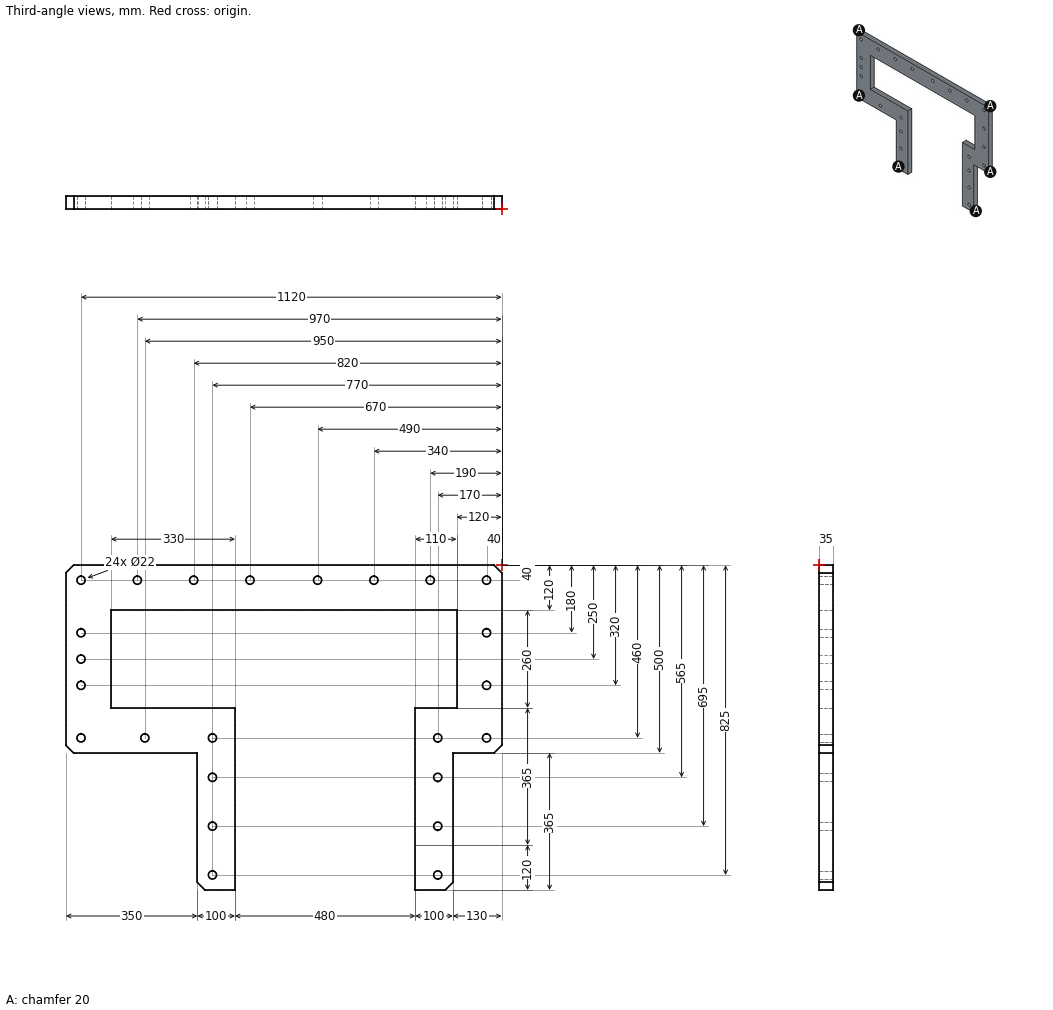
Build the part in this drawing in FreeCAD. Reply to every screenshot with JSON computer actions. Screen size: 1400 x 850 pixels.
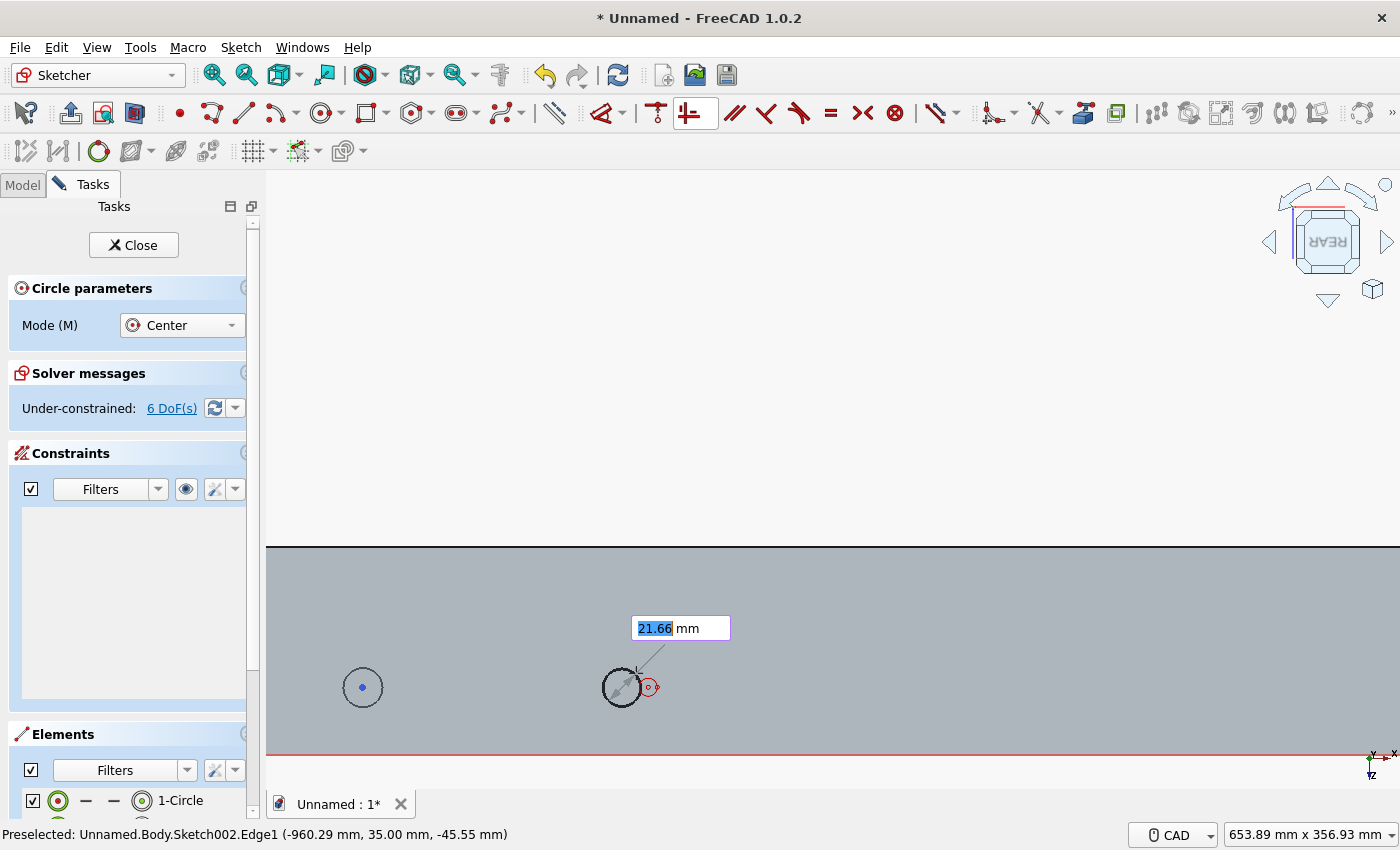
{"action": "left_click", "coordinate": [636, 672]}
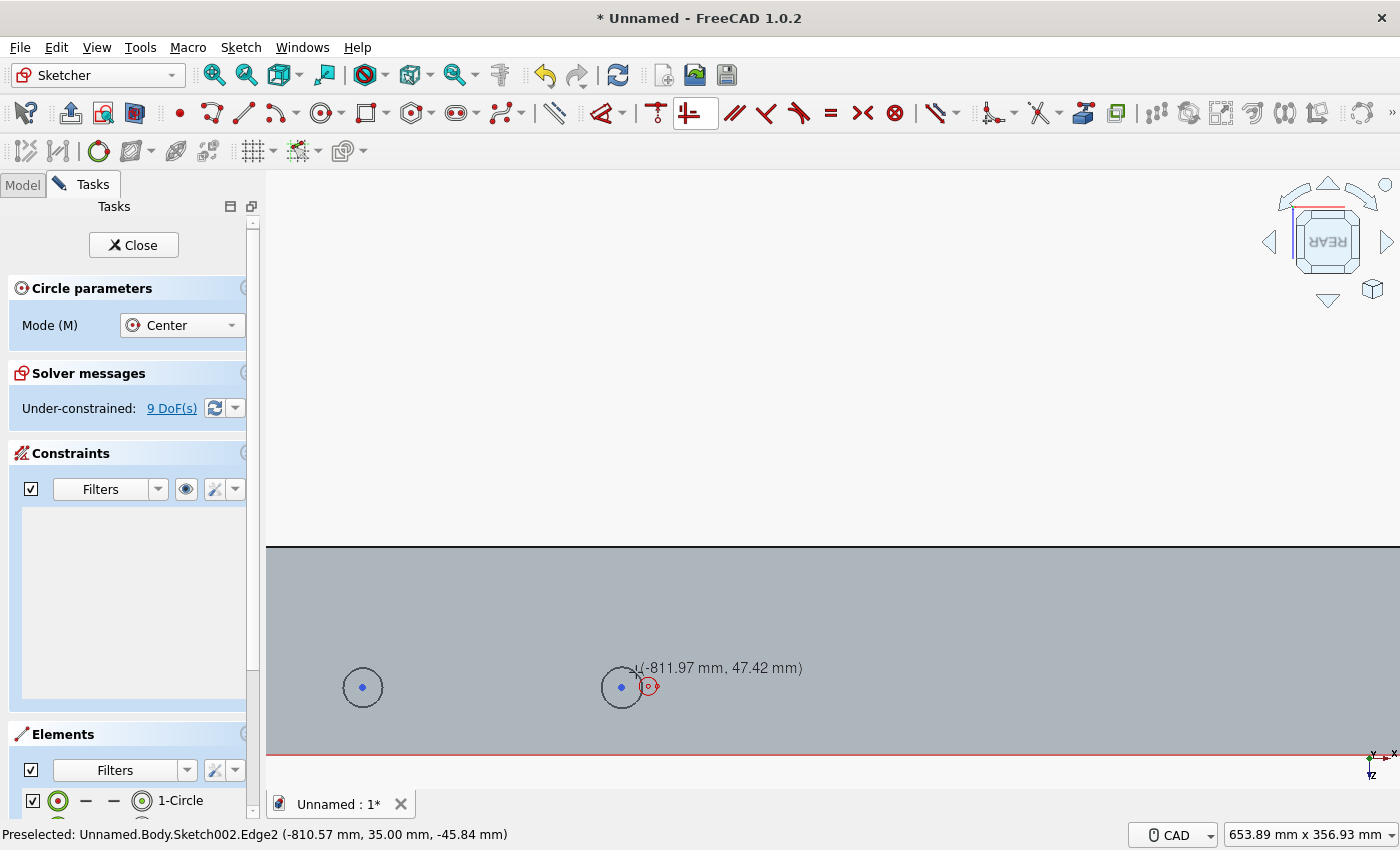
{"action": "scroll", "coordinate": [636, 673], "scroll_direction": "down", "scroll_amount": 6}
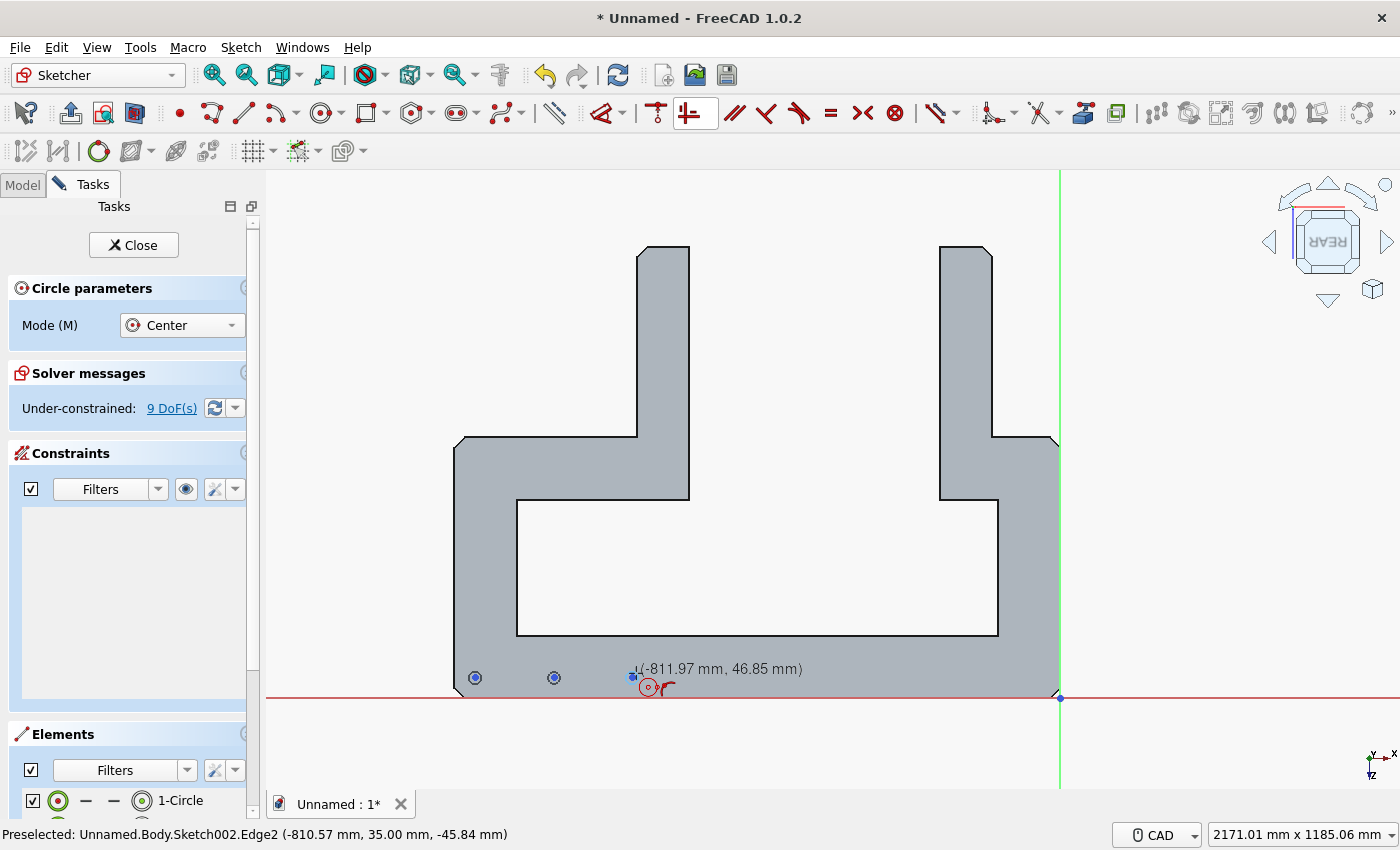
{"action": "left_click", "coordinate": [710, 677]}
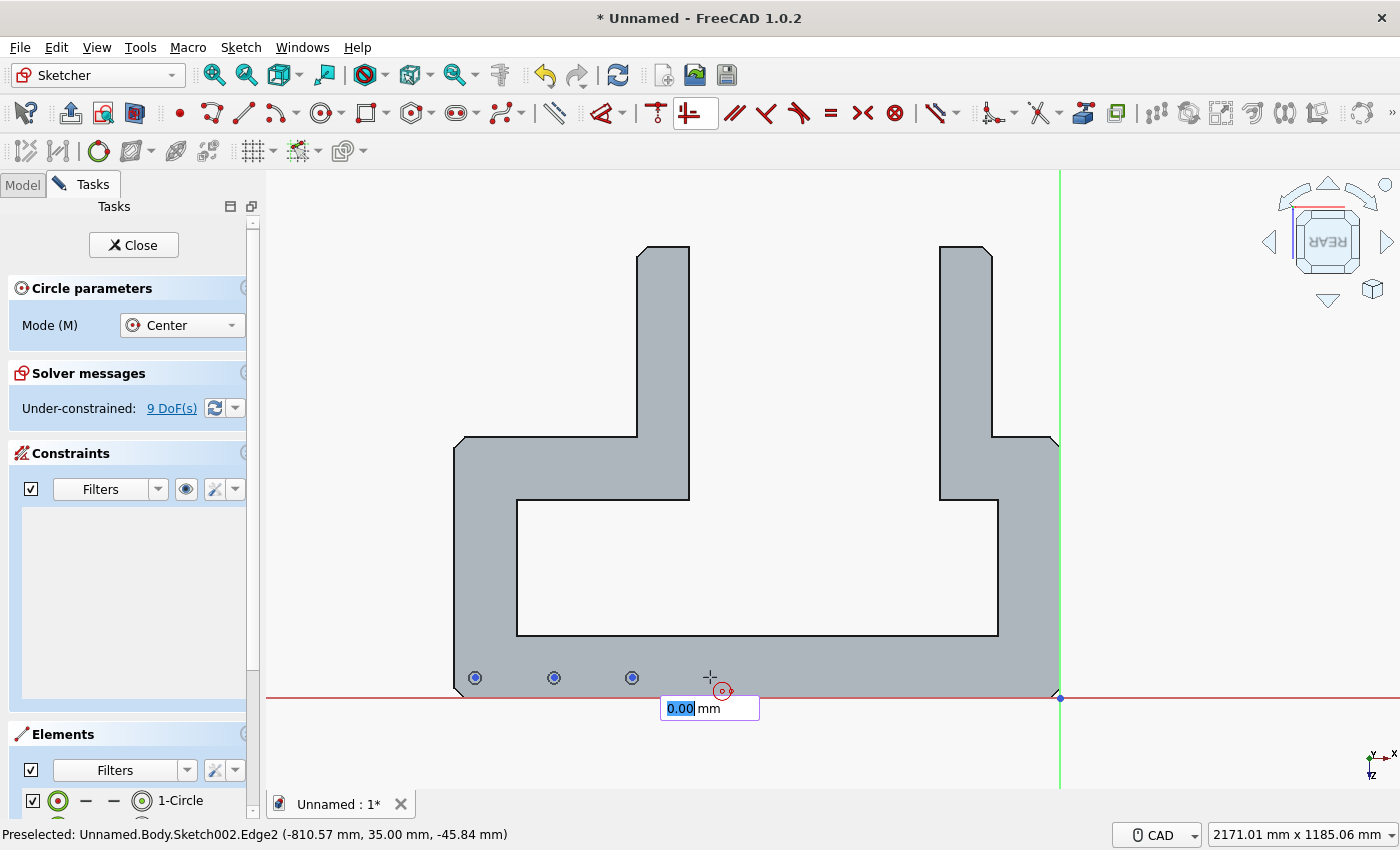
{"action": "scroll", "coordinate": [714, 673], "scroll_direction": "up", "scroll_amount": 6}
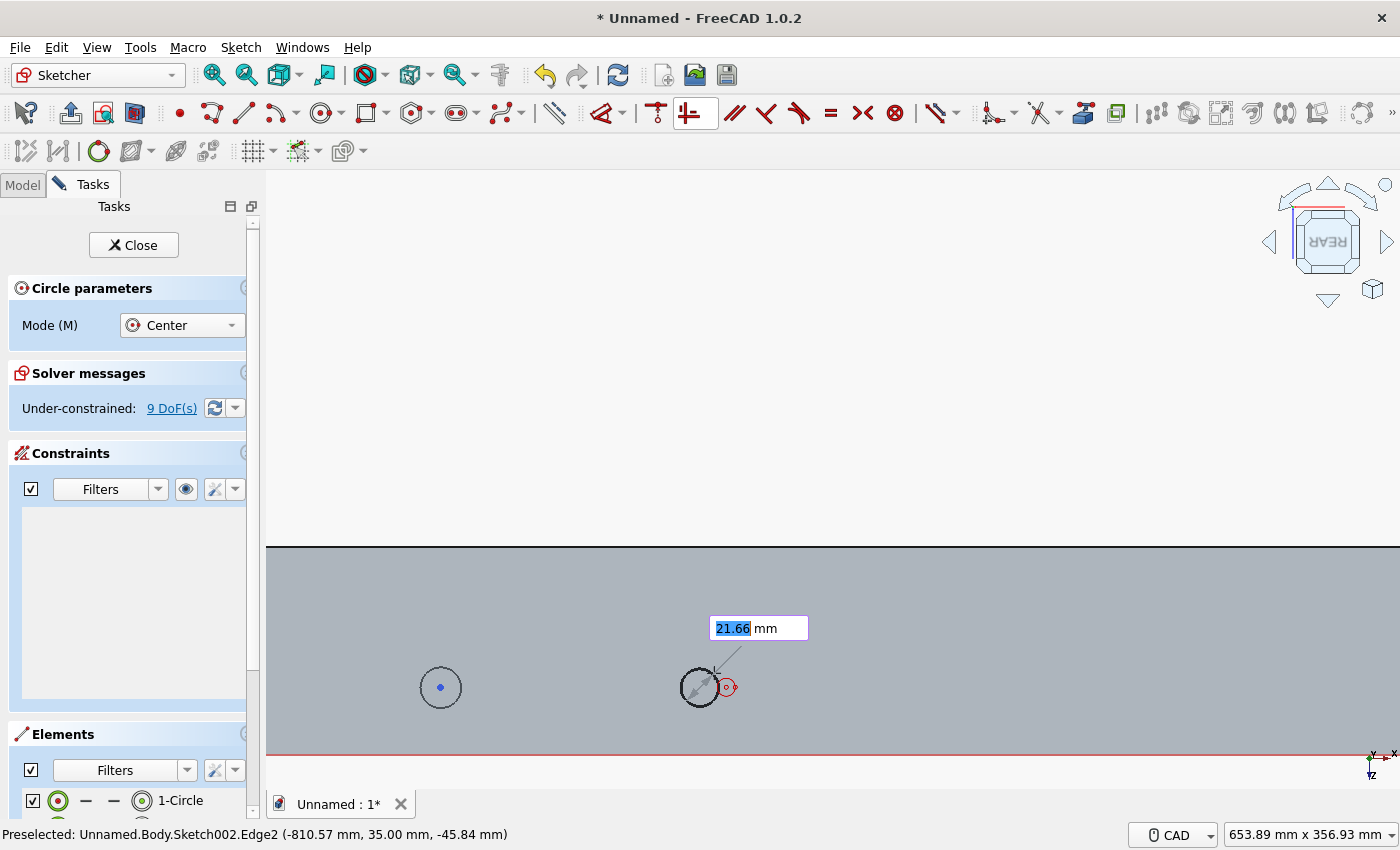
{"action": "left_click", "coordinate": [715, 672]}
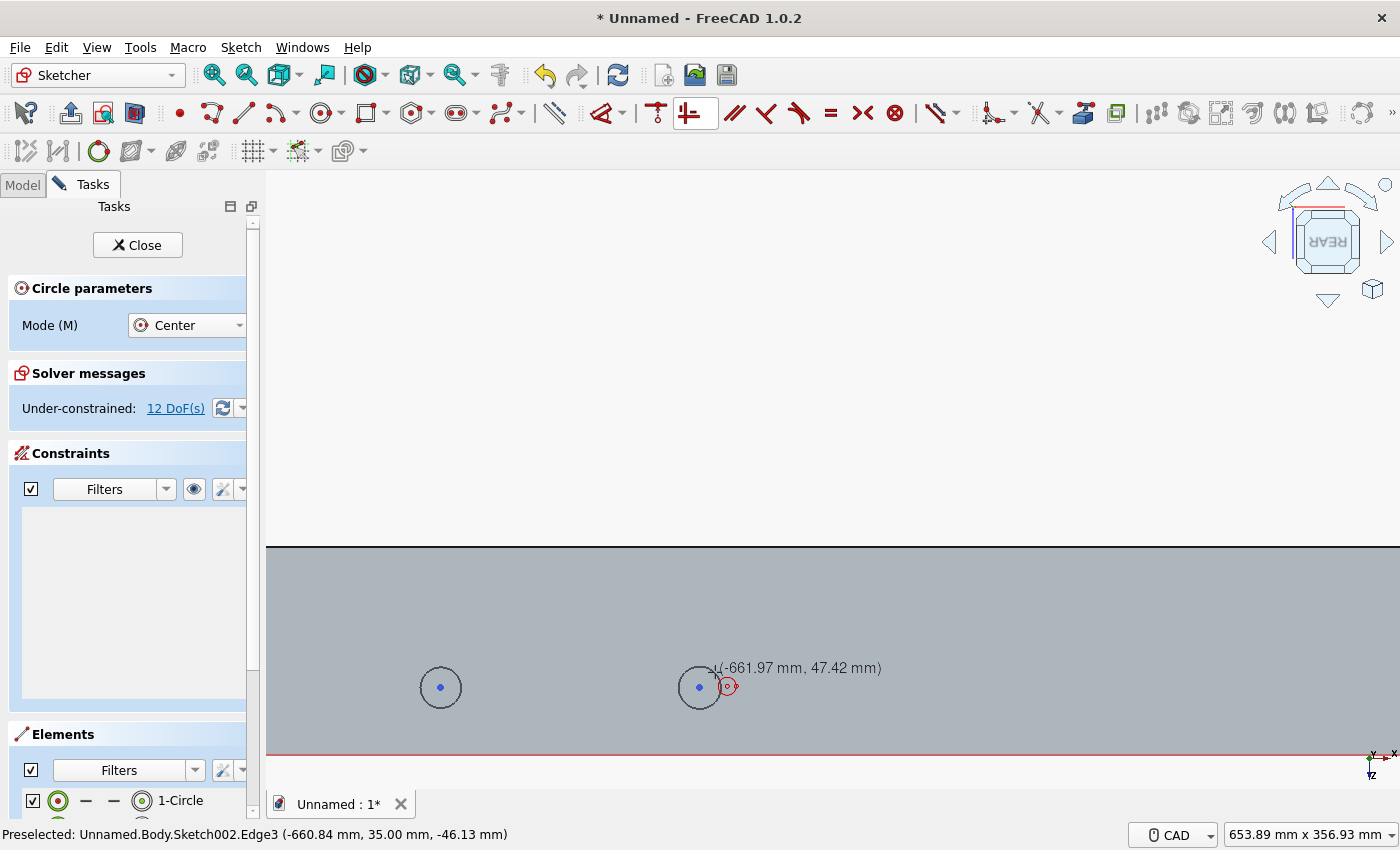
{"action": "scroll", "coordinate": [714, 673], "scroll_direction": "down", "scroll_amount": 6}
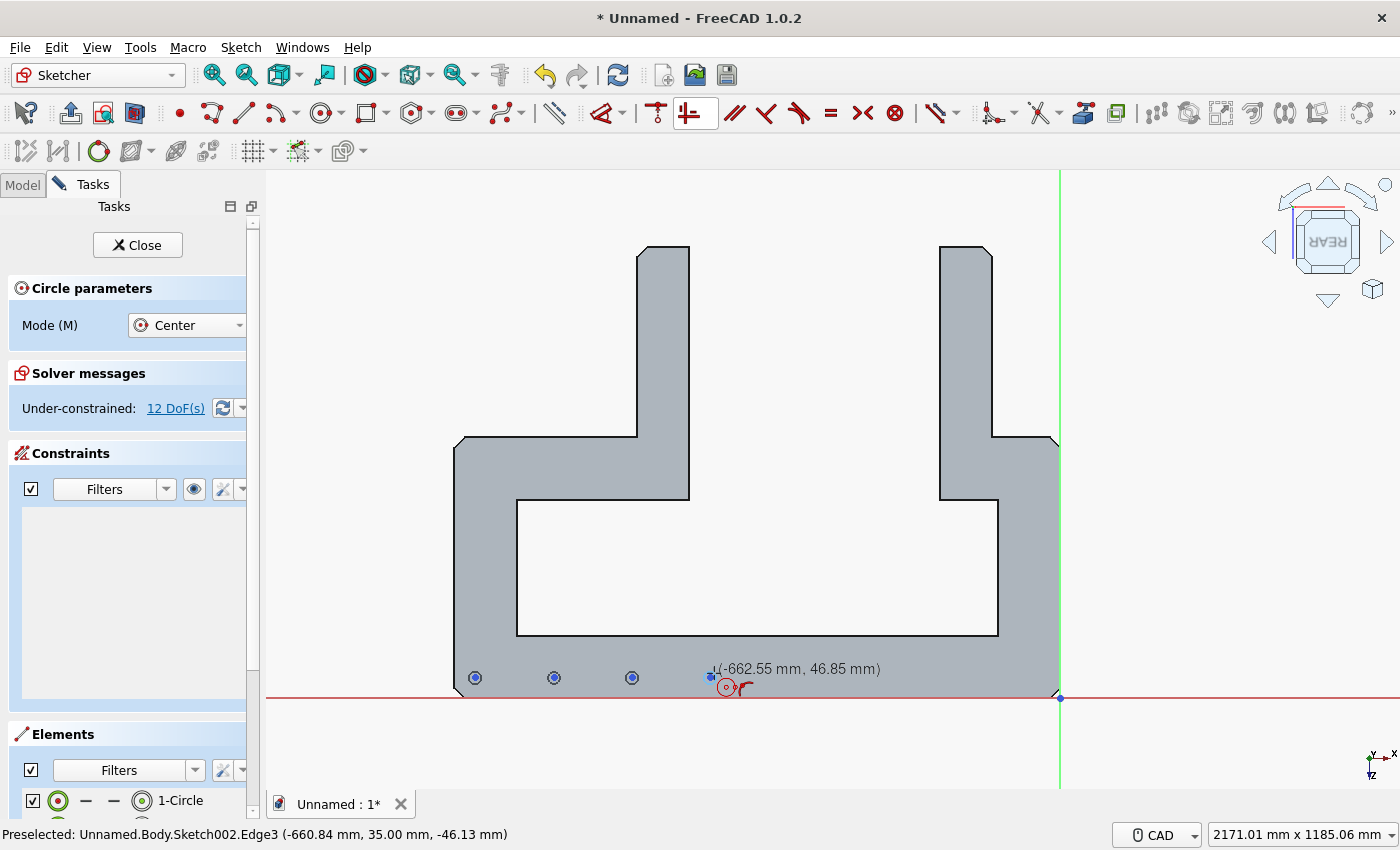
{"action": "left_click", "coordinate": [804, 677]}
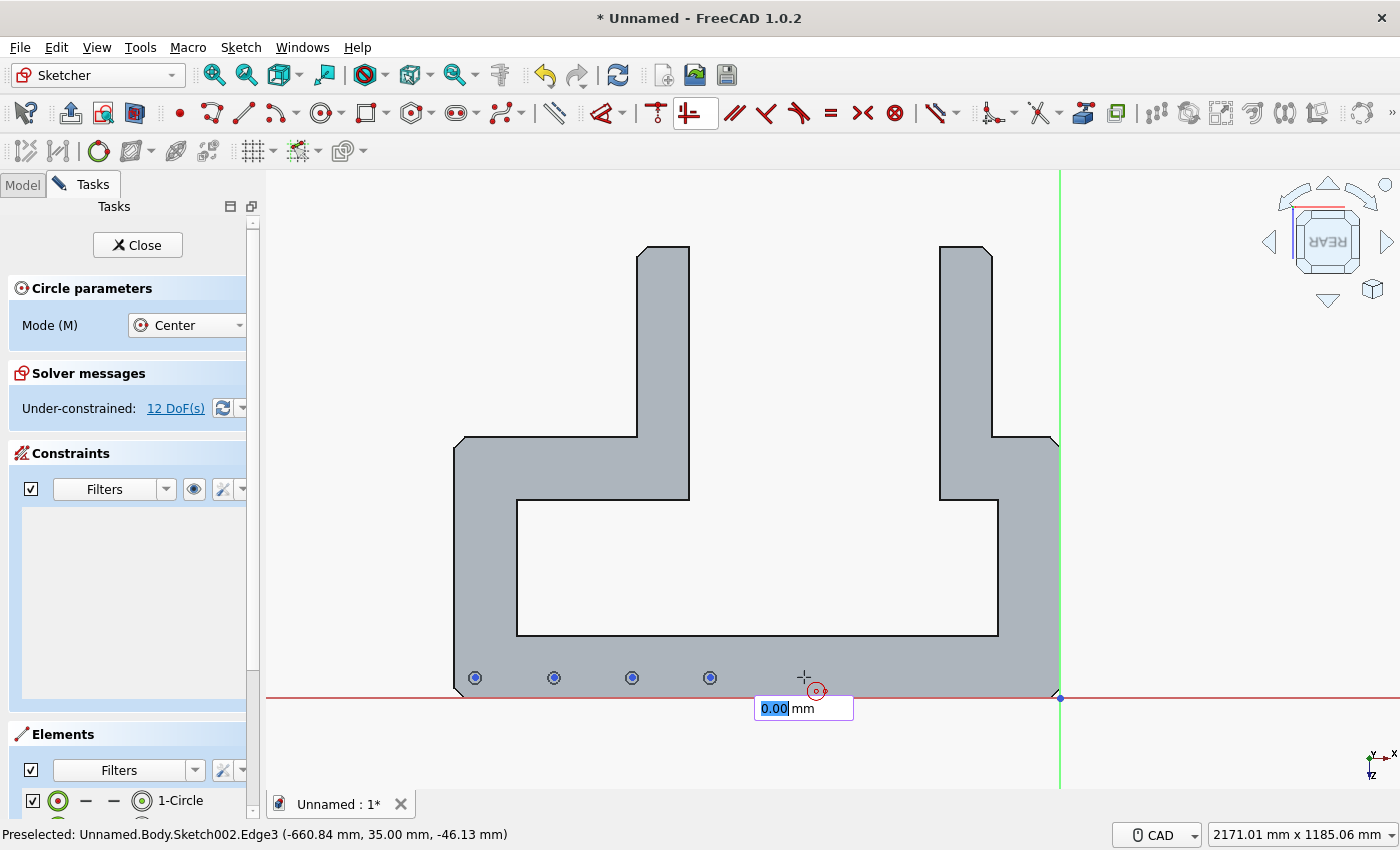
{"action": "scroll", "coordinate": [808, 673], "scroll_direction": "up", "scroll_amount": 6}